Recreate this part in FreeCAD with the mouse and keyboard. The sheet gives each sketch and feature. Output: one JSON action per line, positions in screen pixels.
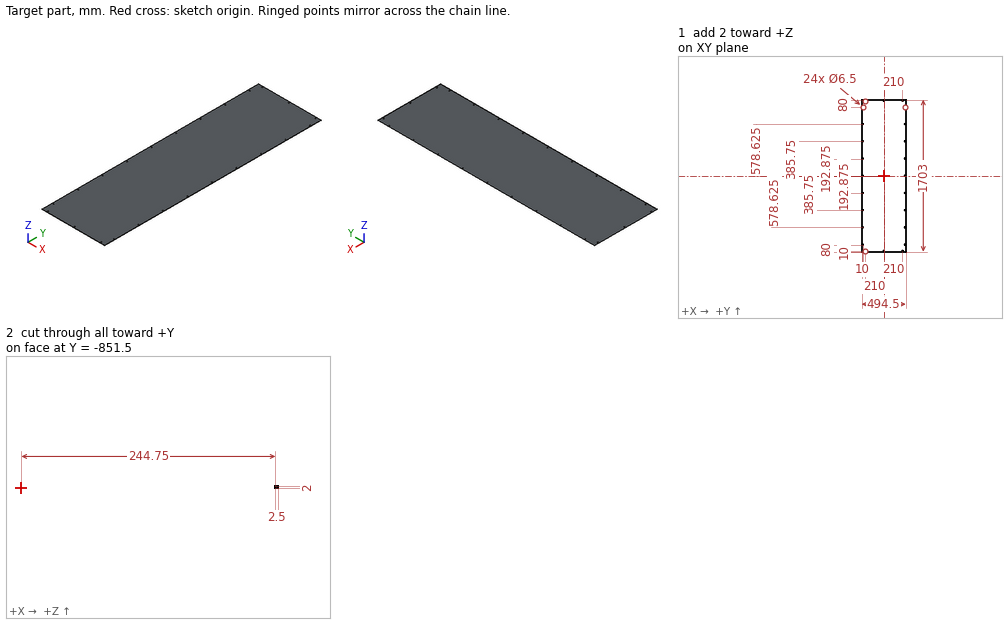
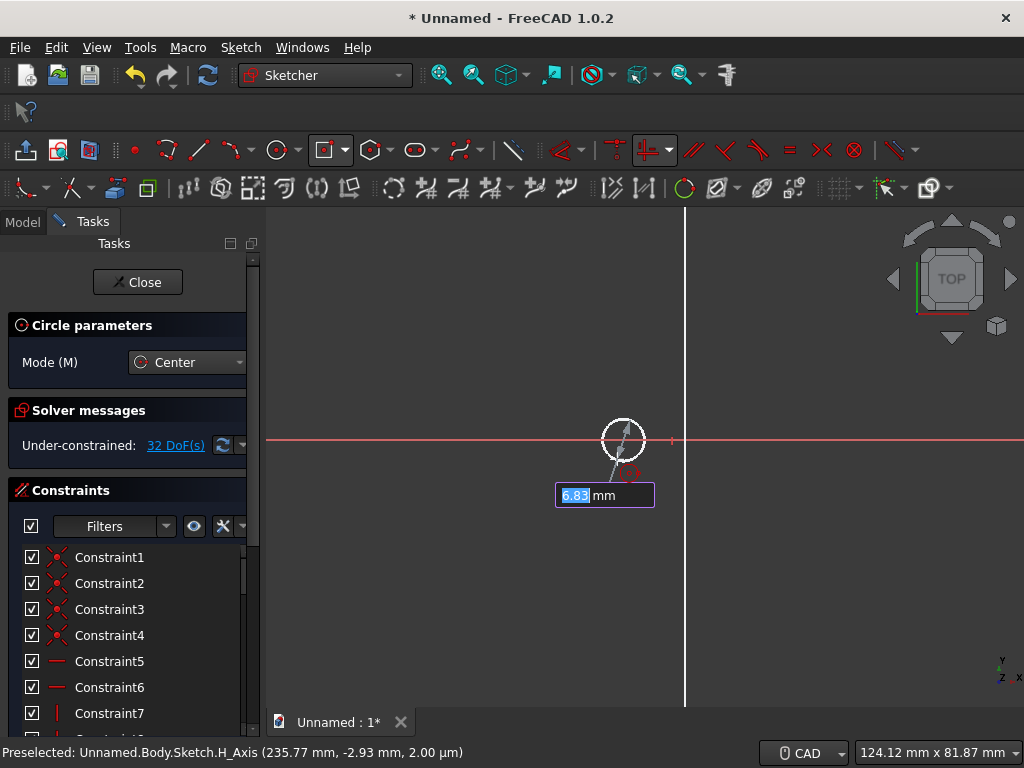
{"action": "type", "text": "6.5"}
{"action": "key", "text": "Return"}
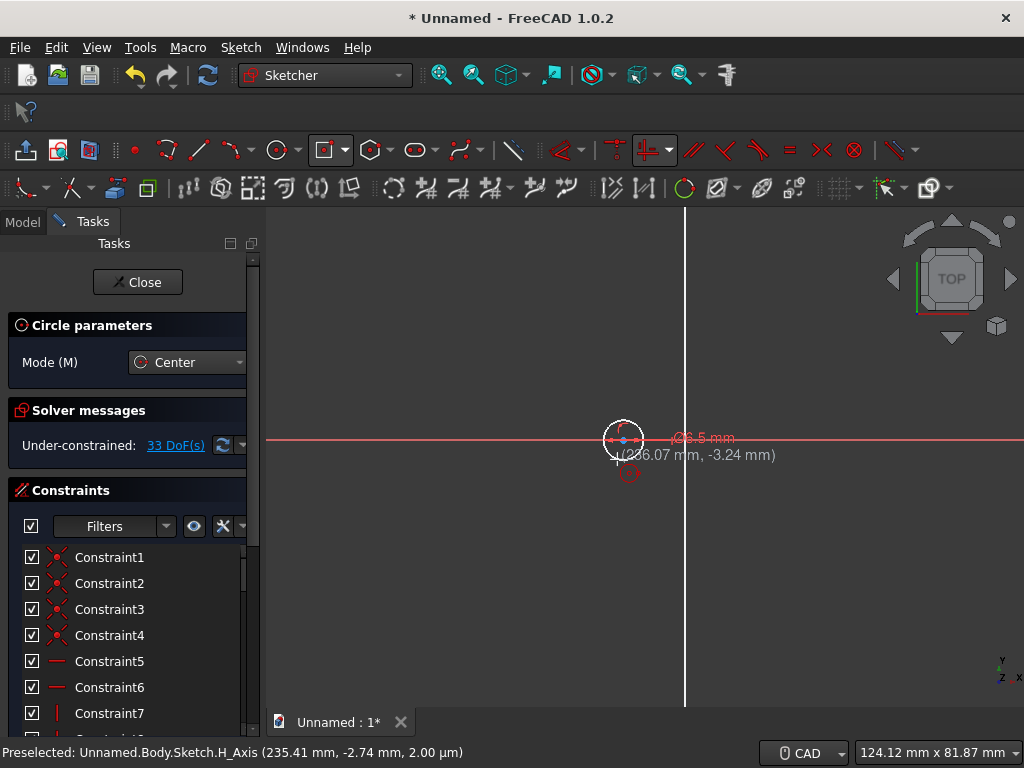
{"action": "scroll", "coordinate": [625, 458], "scroll_direction": "down", "scroll_amount": 17}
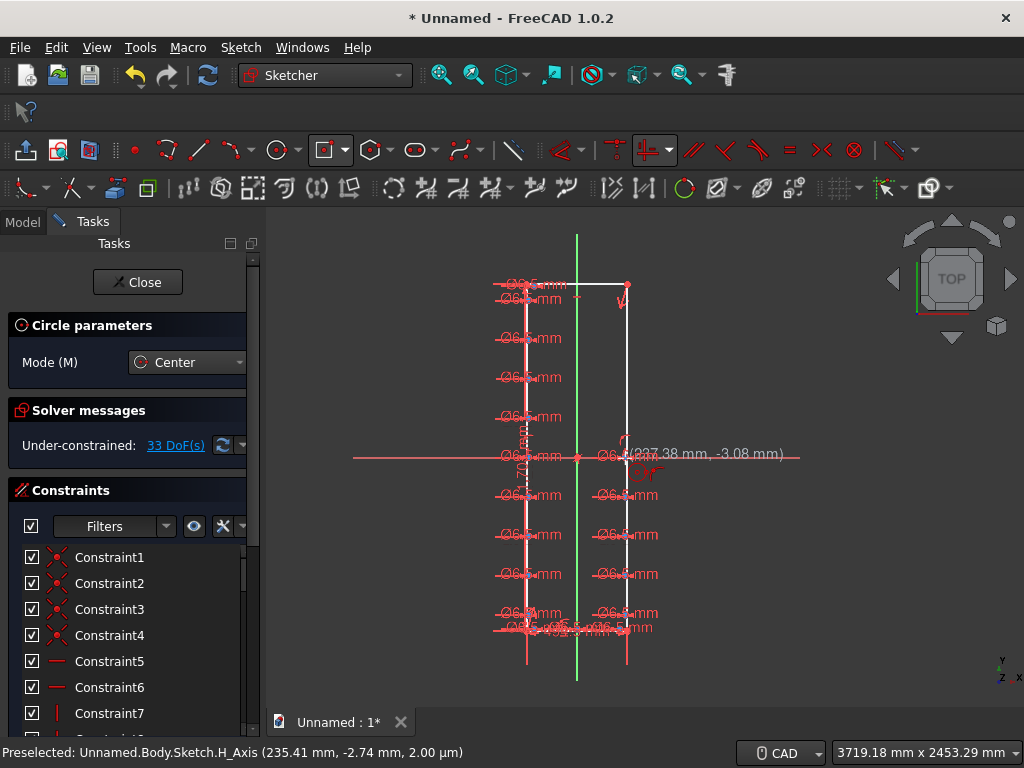
{"action": "scroll", "coordinate": [625, 419], "scroll_direction": "up", "scroll_amount": 18}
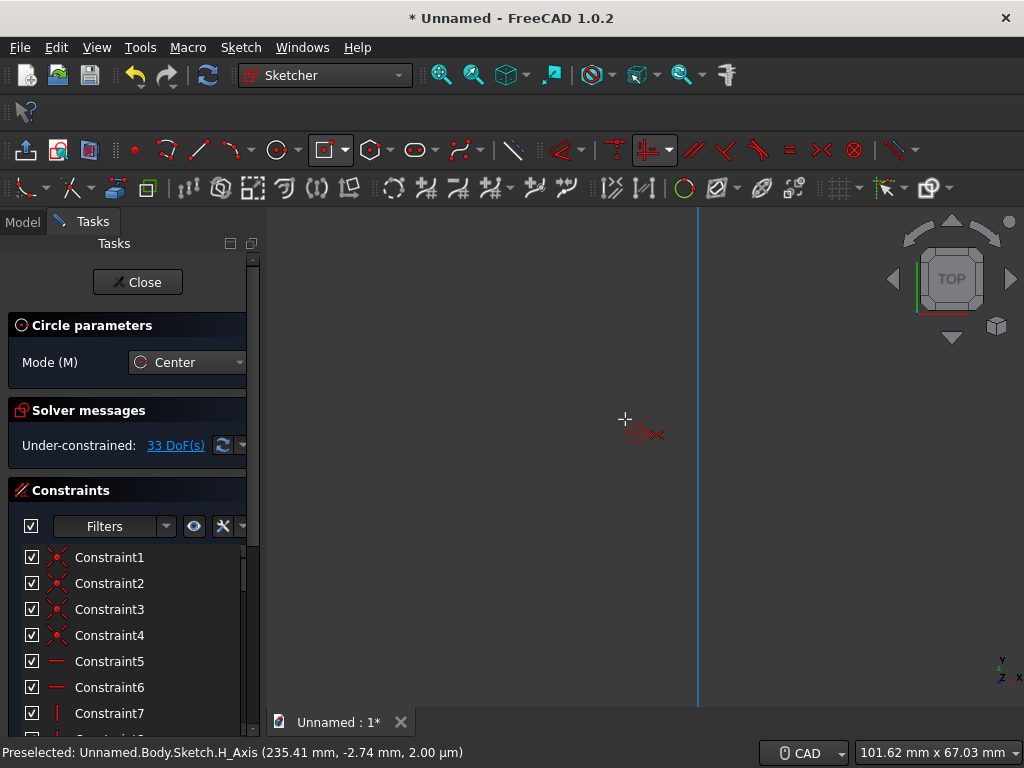
{"action": "scroll", "coordinate": [625, 419], "scroll_direction": "down", "scroll_amount": 18}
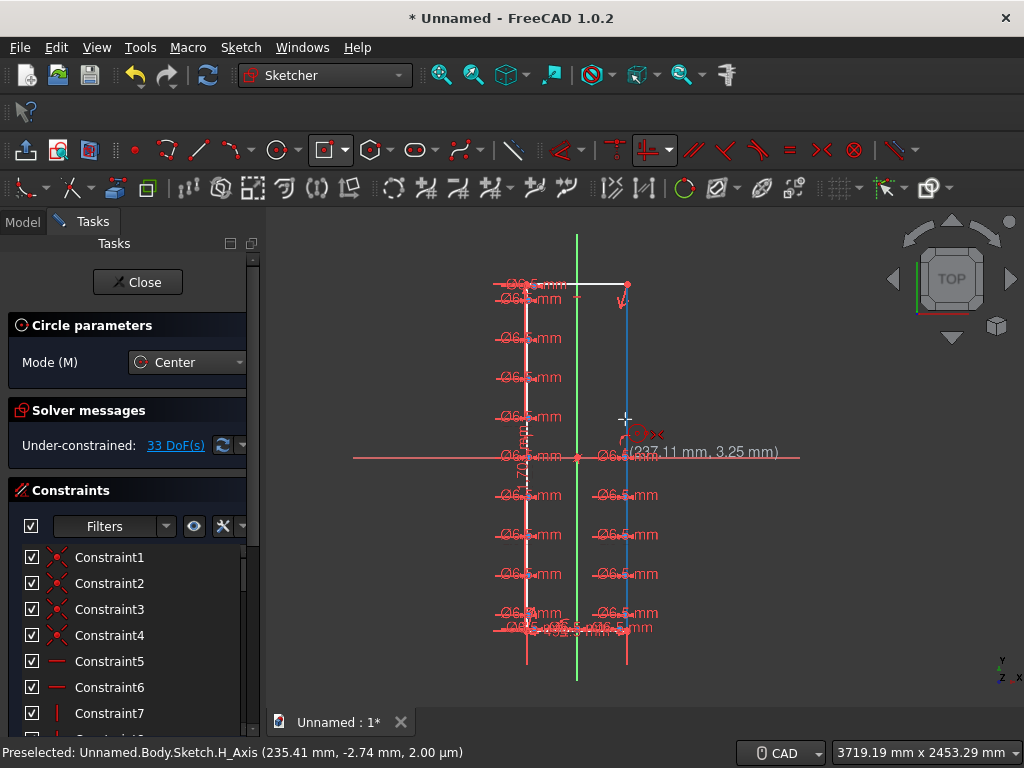
{"action": "scroll", "coordinate": [625, 419], "scroll_direction": "up", "scroll_amount": 11}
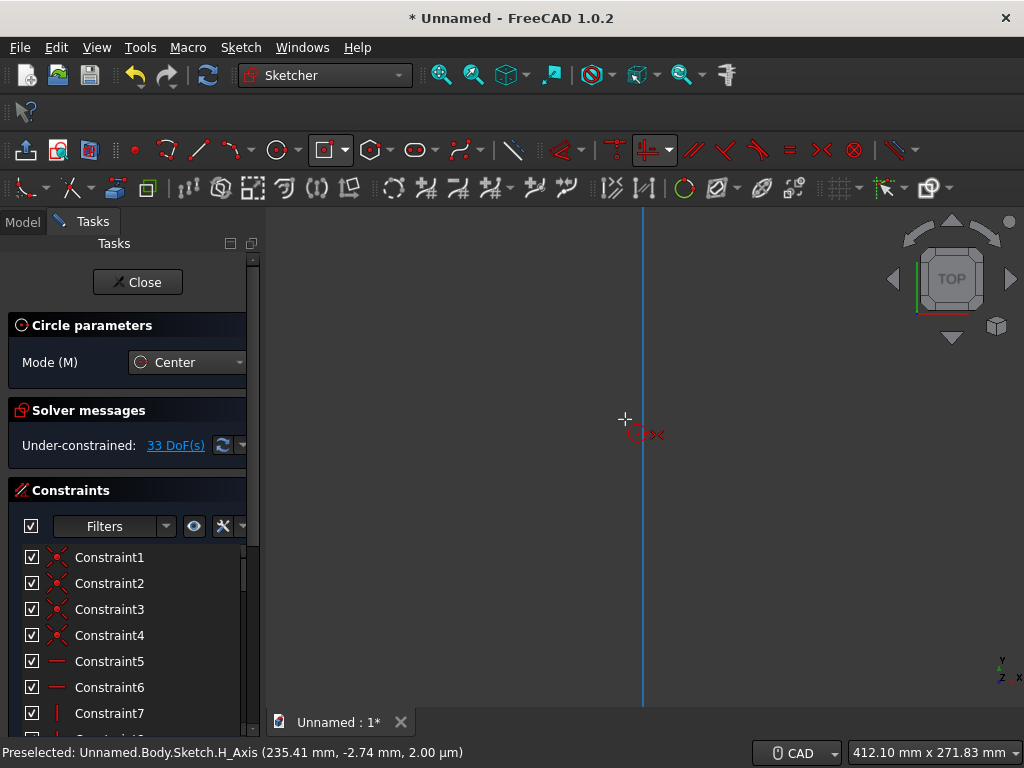
{"action": "left_click", "coordinate": [625, 412]}
{"action": "mouse_move", "coordinate": [629, 408]}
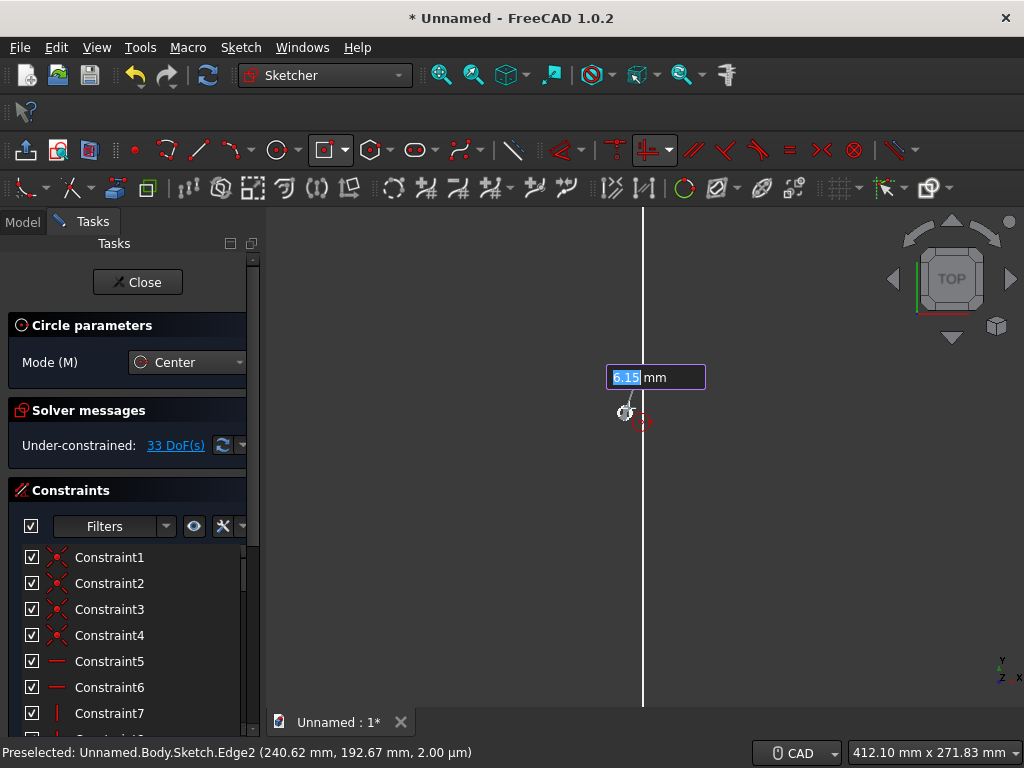
{"action": "type", "text": "6.5"}
{"action": "key", "text": "Return"}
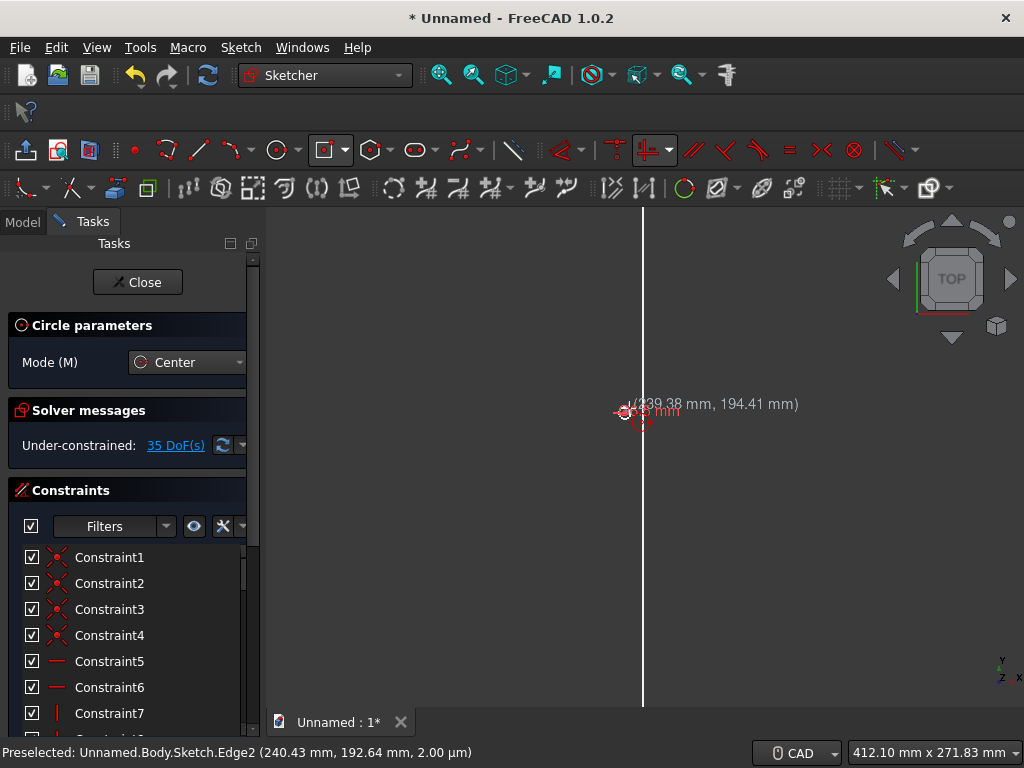
{"action": "scroll", "coordinate": [615, 426], "scroll_direction": "down", "scroll_amount": 12}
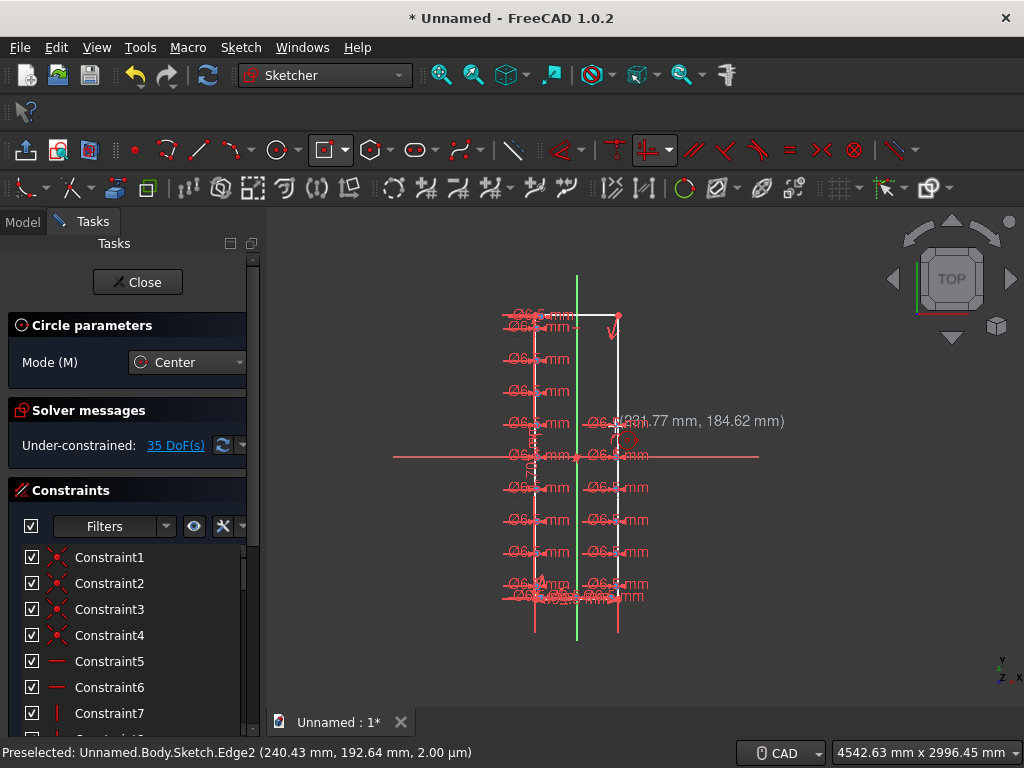
{"action": "scroll", "coordinate": [616, 393], "scroll_direction": "up", "scroll_amount": 19}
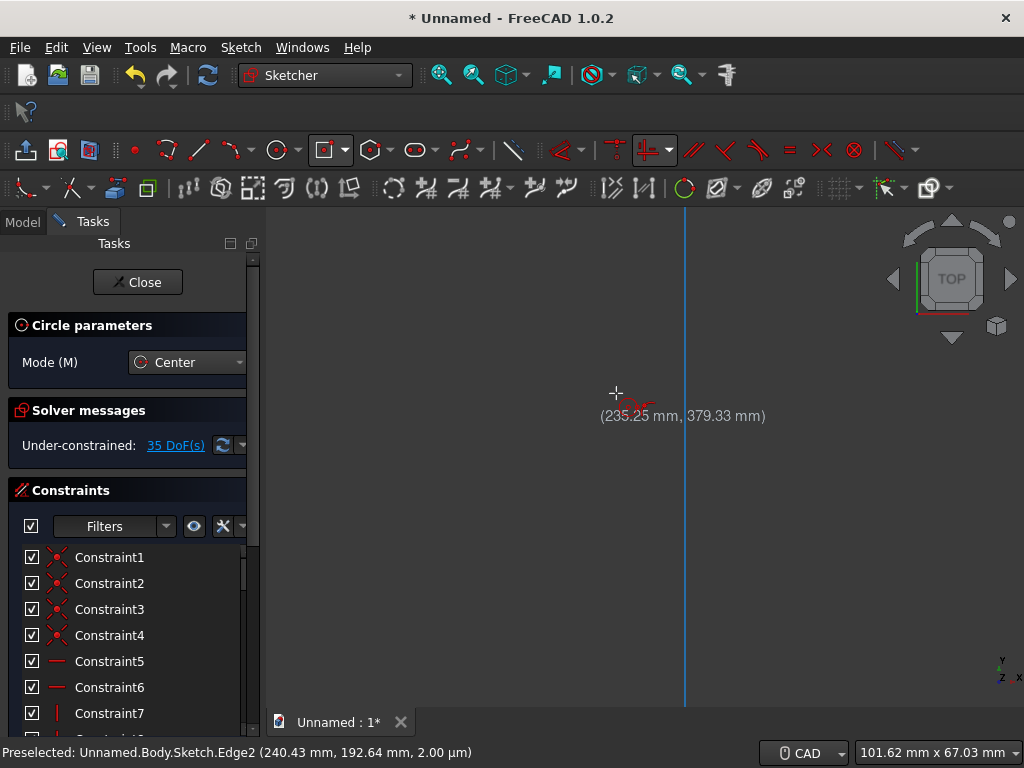
{"action": "scroll", "coordinate": [625, 379], "scroll_direction": "down", "scroll_amount": 18}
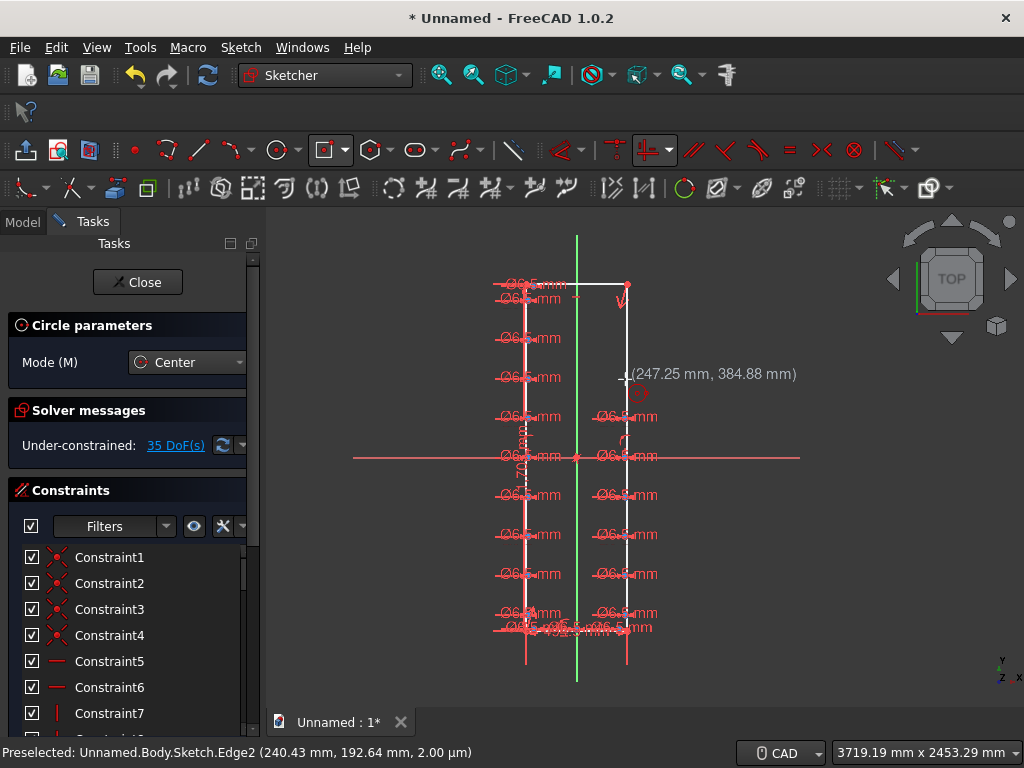
{"action": "scroll", "coordinate": [625, 379], "scroll_direction": "up", "scroll_amount": 11}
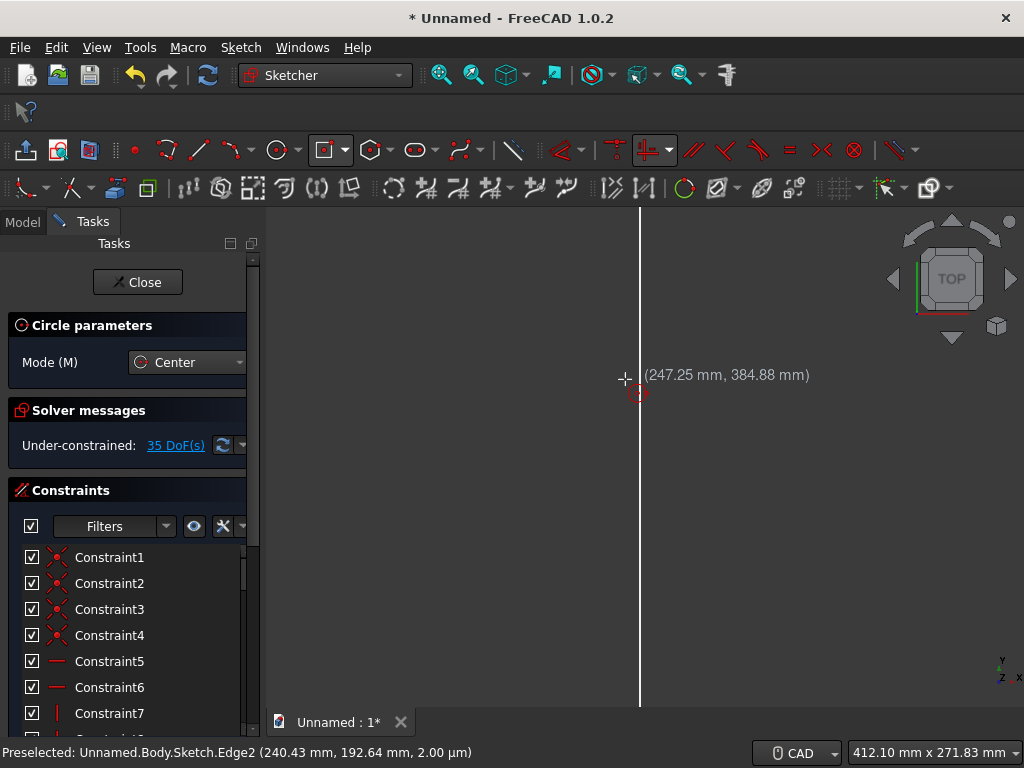
{"action": "left_click", "coordinate": [622, 378]}
{"action": "mouse_move", "coordinate": [626, 374]}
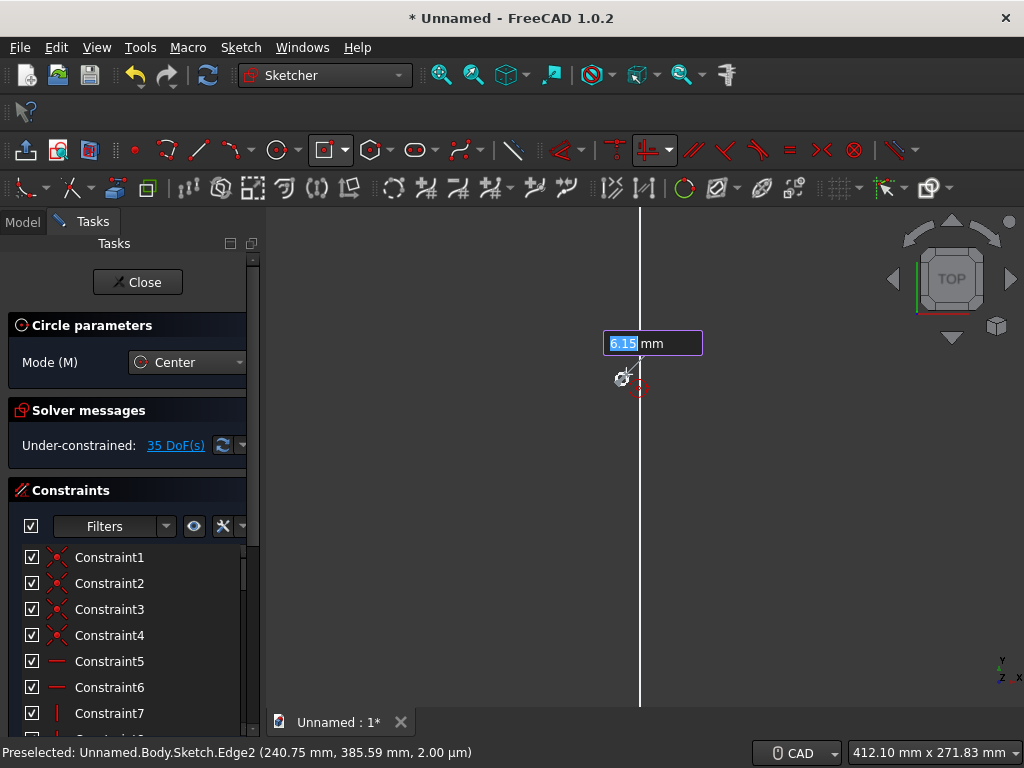
{"action": "type", "text": "6.5"}
{"action": "key", "text": "Return"}